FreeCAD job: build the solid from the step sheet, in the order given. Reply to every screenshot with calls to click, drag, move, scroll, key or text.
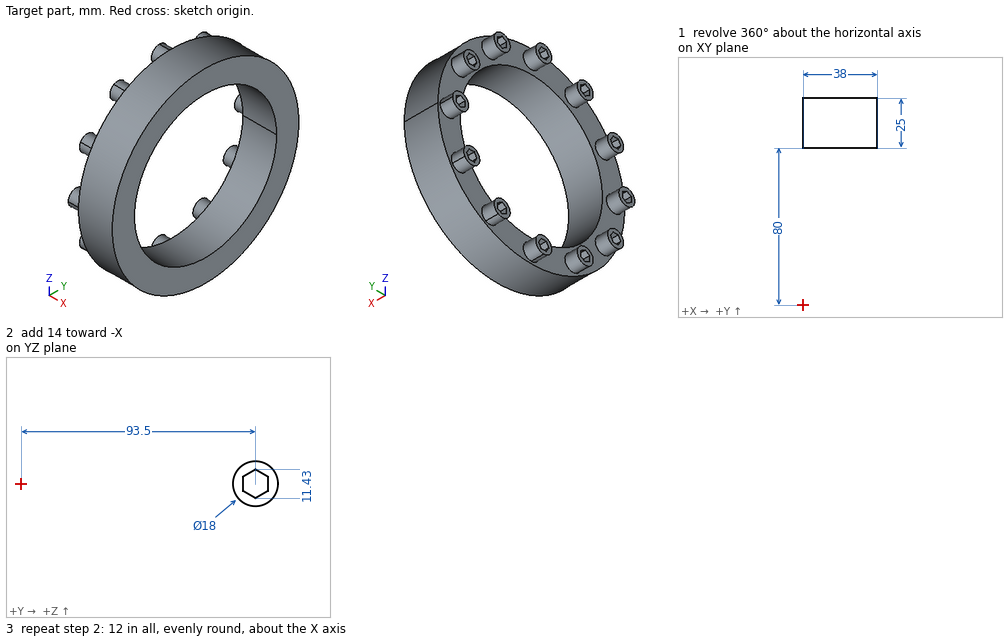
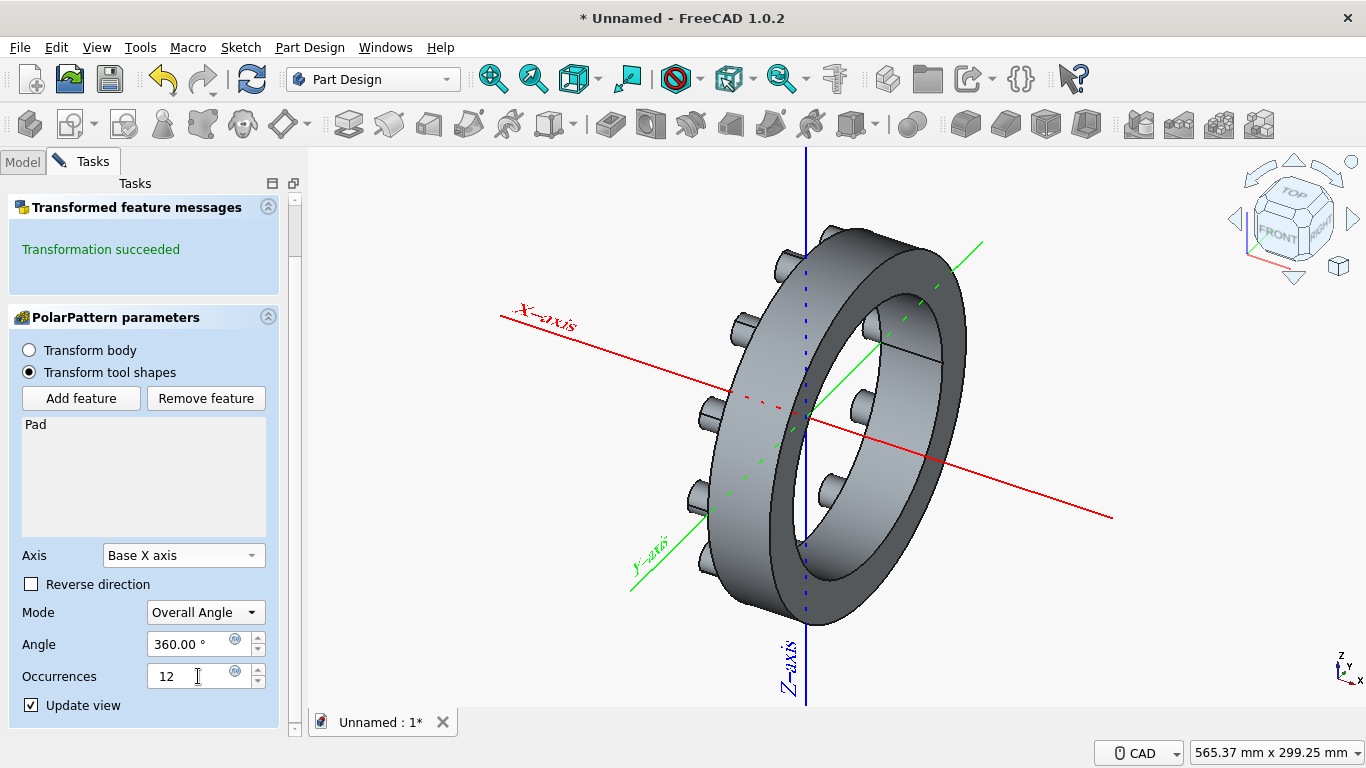
scroll(295, 464, up, 2)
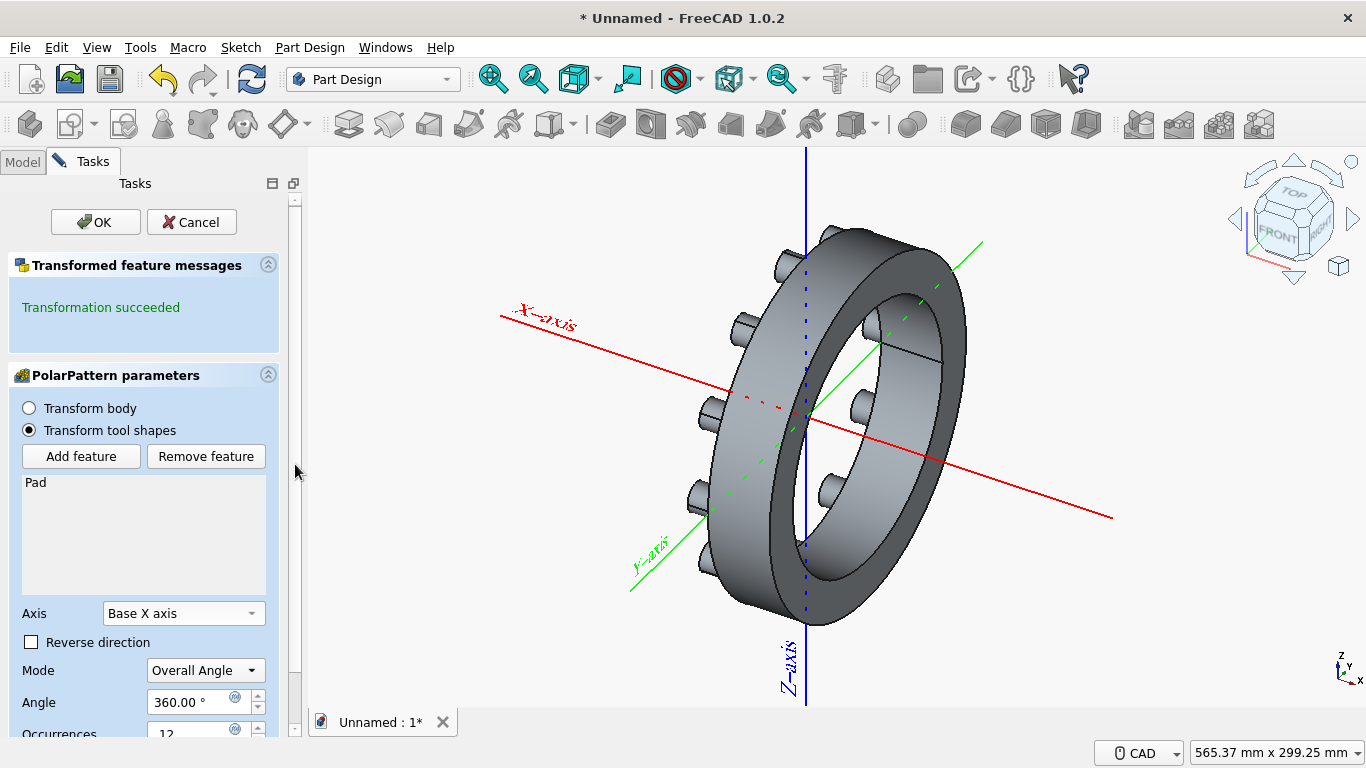
click(96, 222)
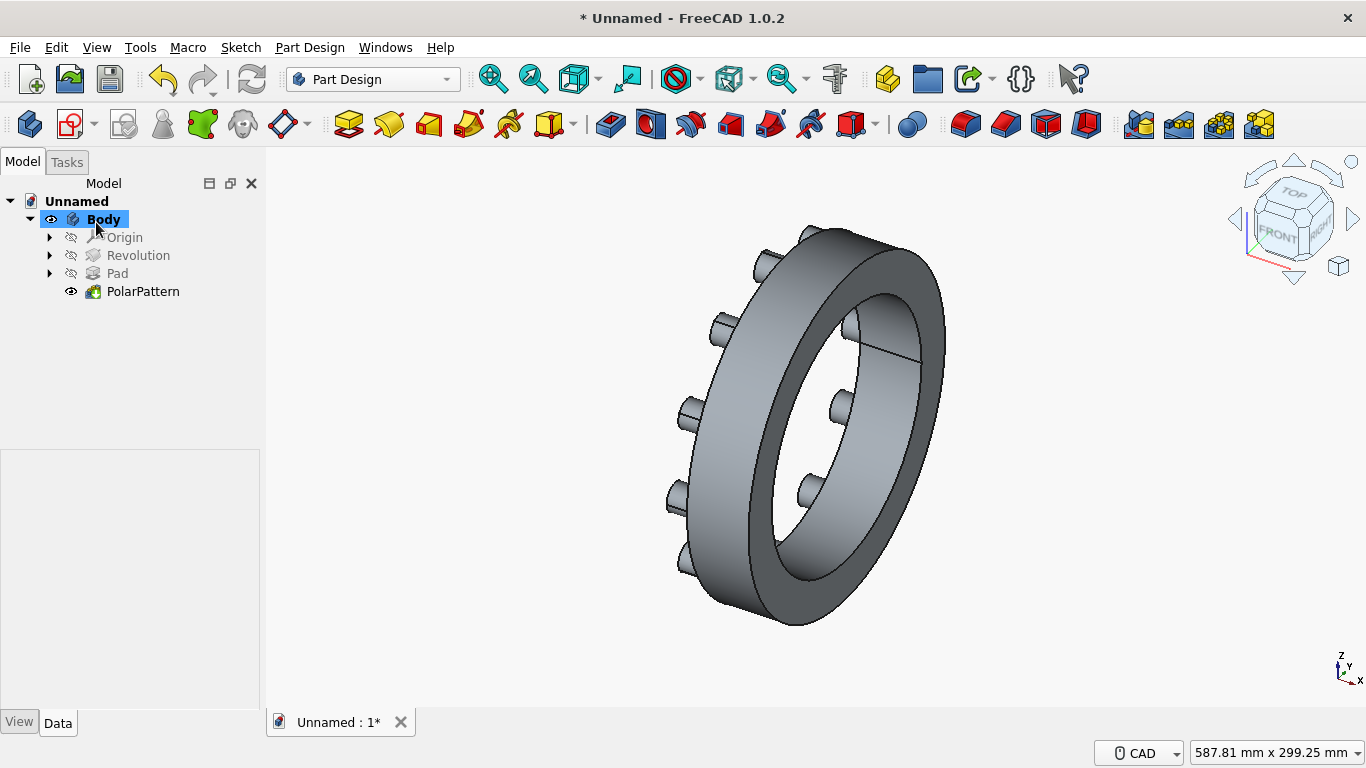
key(0)